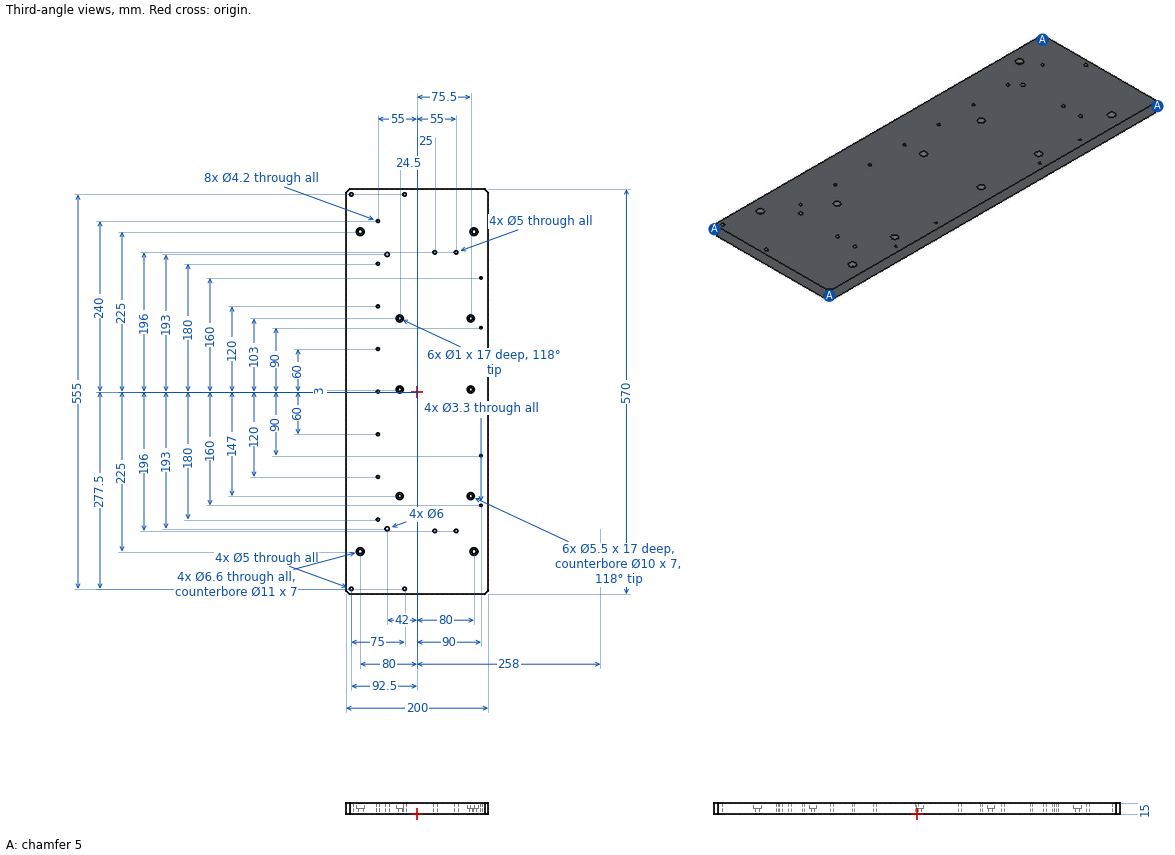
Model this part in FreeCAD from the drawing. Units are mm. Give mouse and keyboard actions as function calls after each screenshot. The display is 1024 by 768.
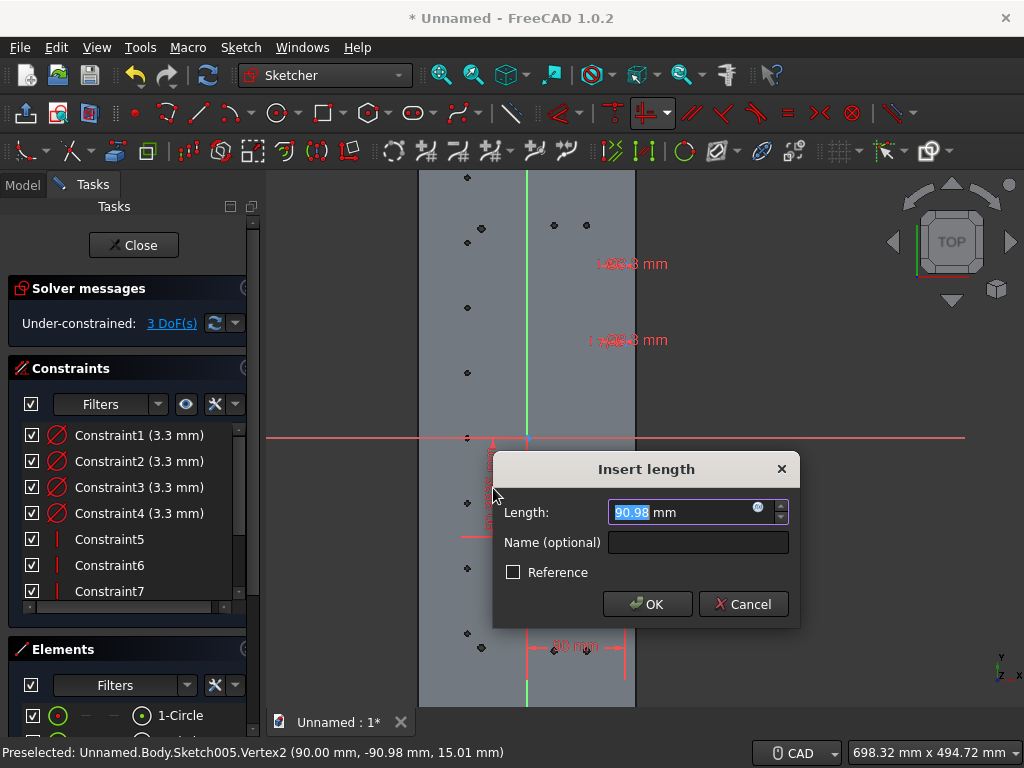
text(90)
key(Return)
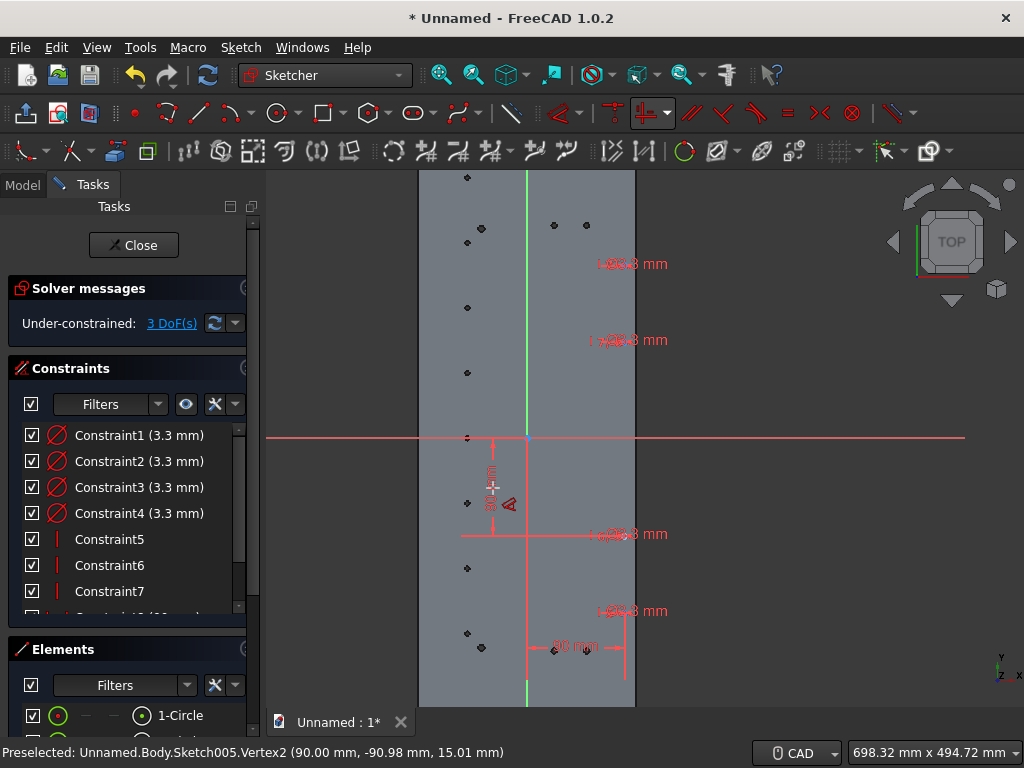
click(625, 342)
click(493, 390)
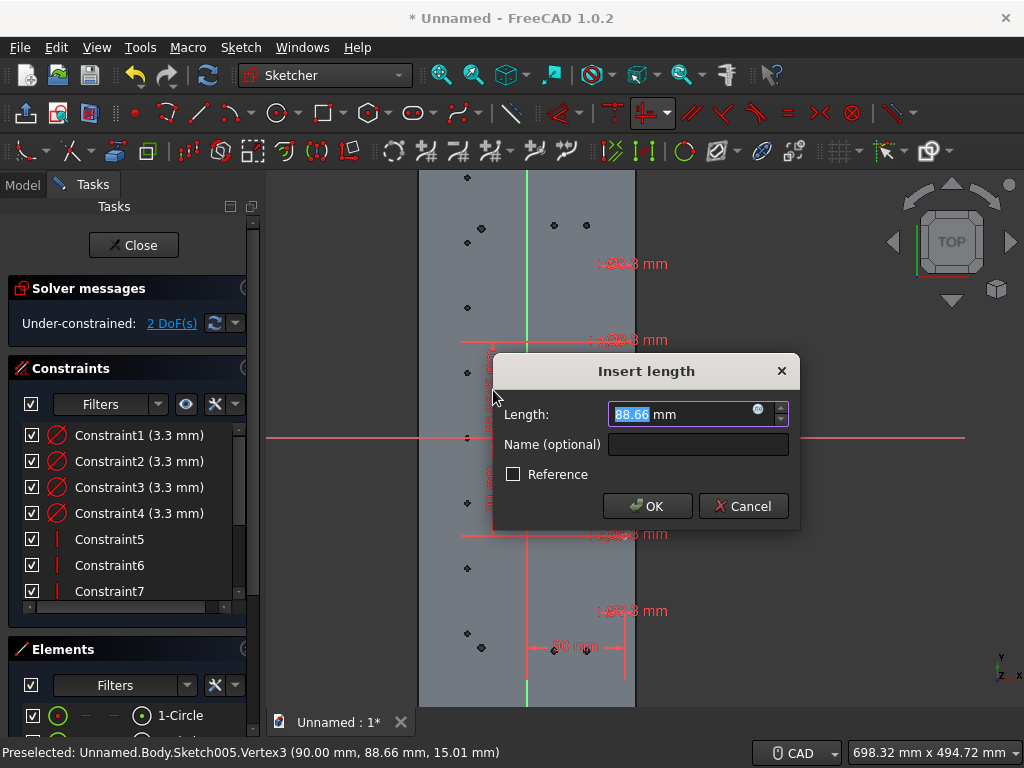
text(90)
key(Return)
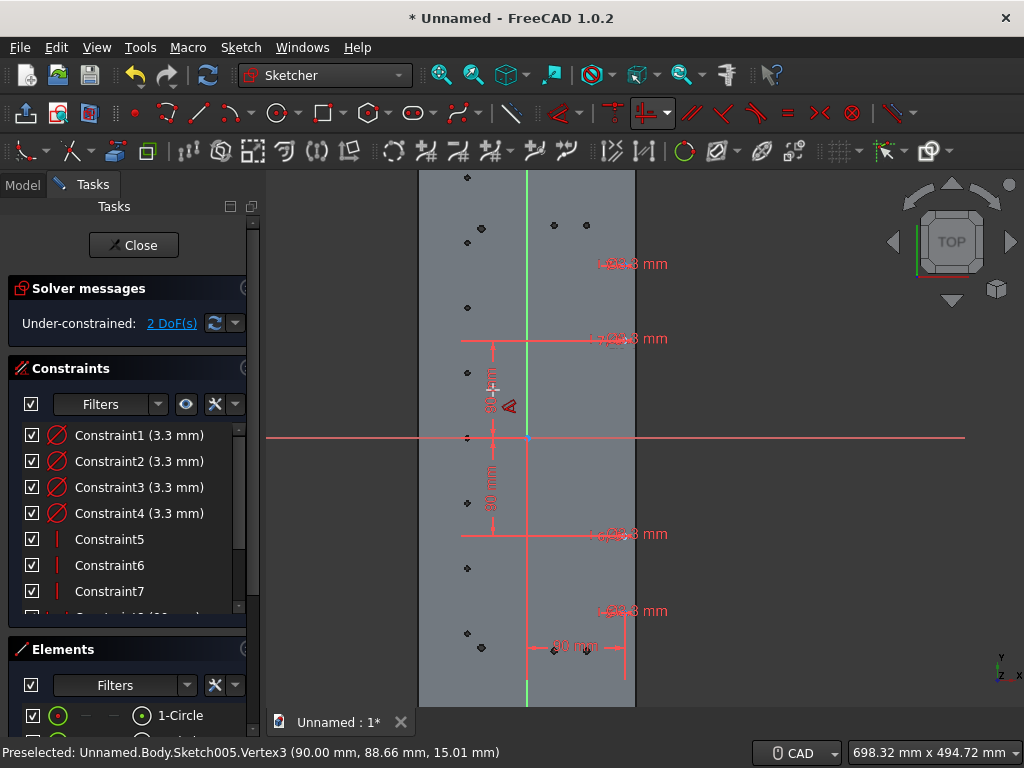
click(625, 613)
click(493, 526)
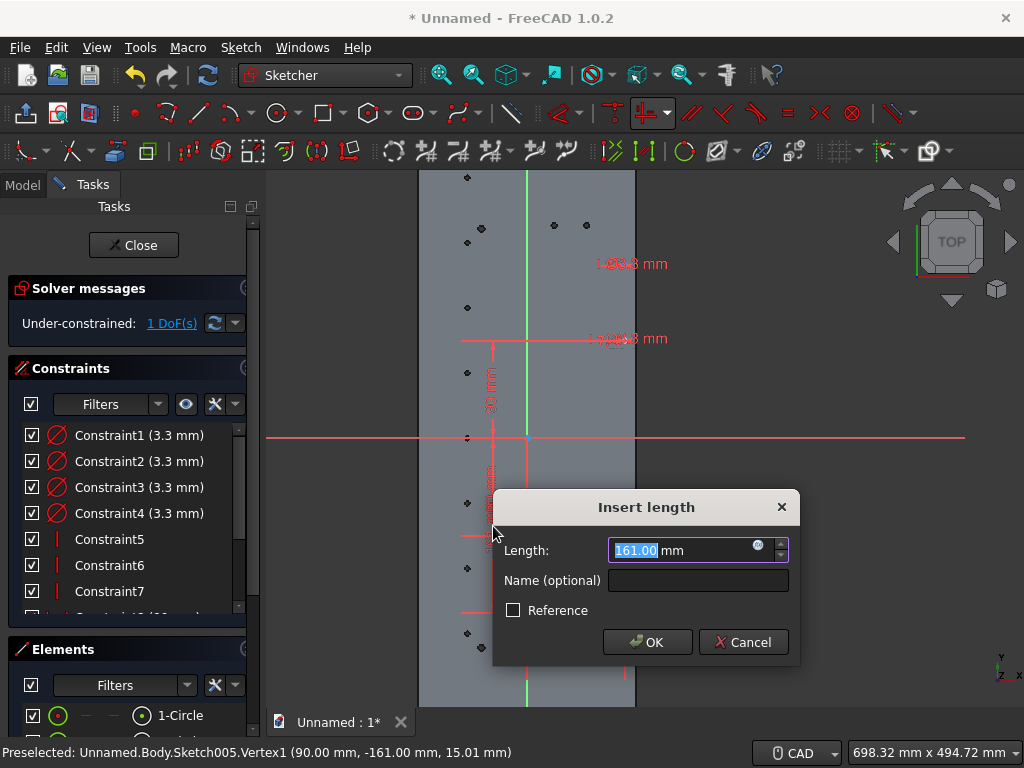
text(160)
key(Return)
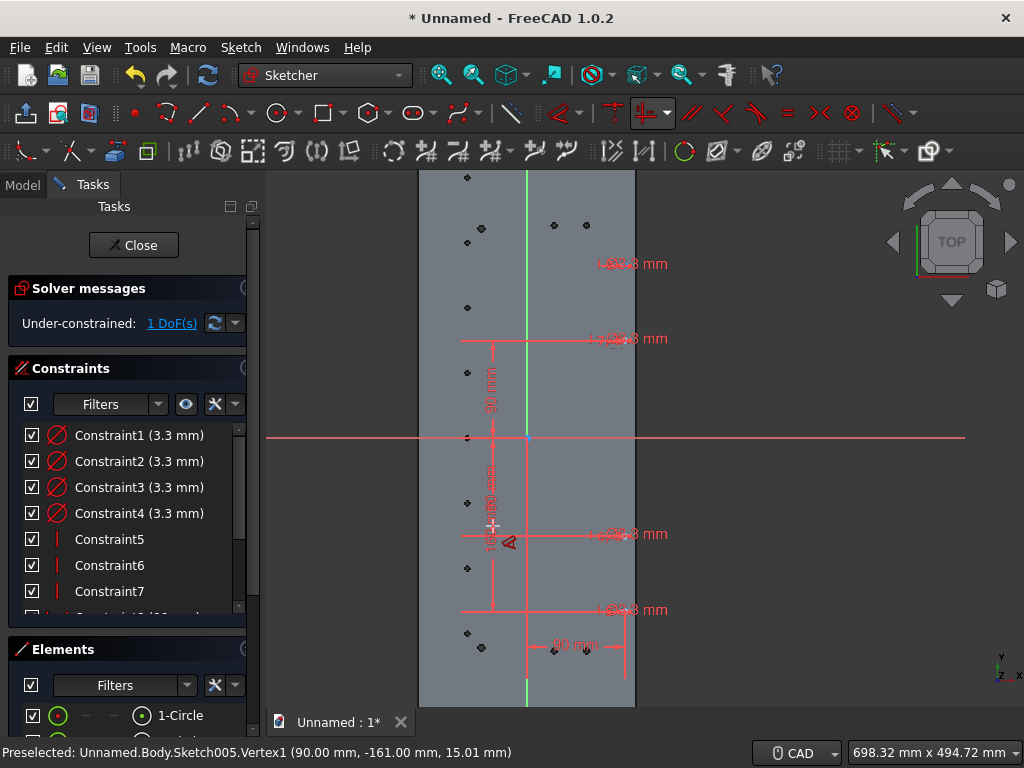
click(625, 266)
click(493, 352)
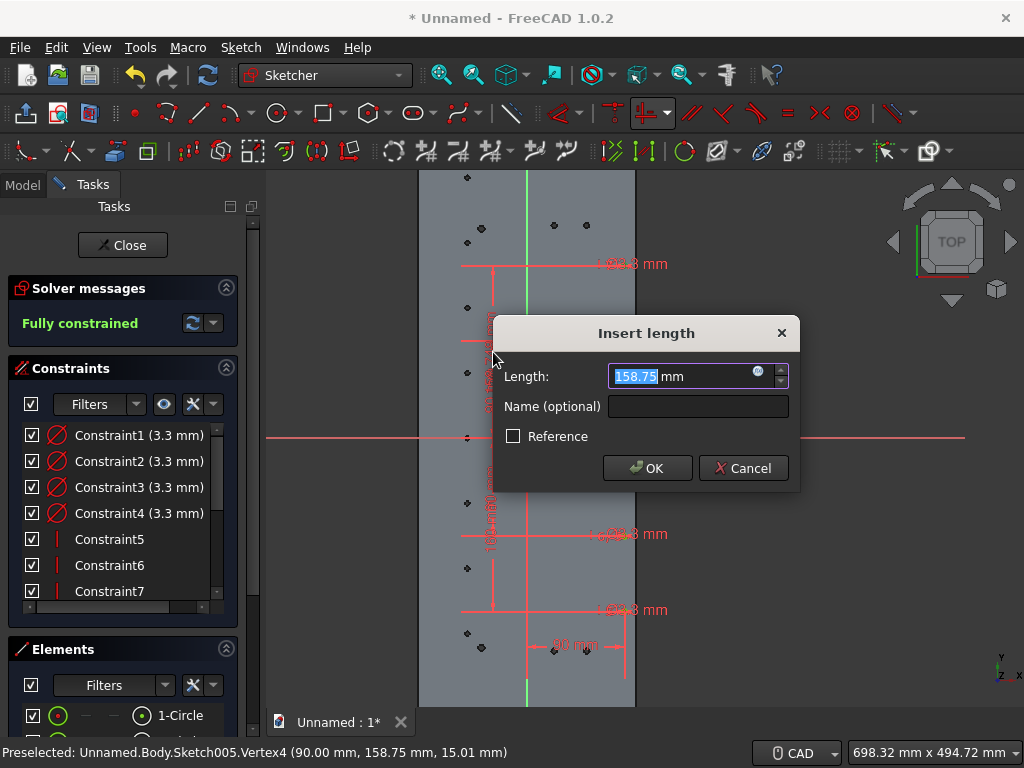
text(160)
key(Return)
key(Escape)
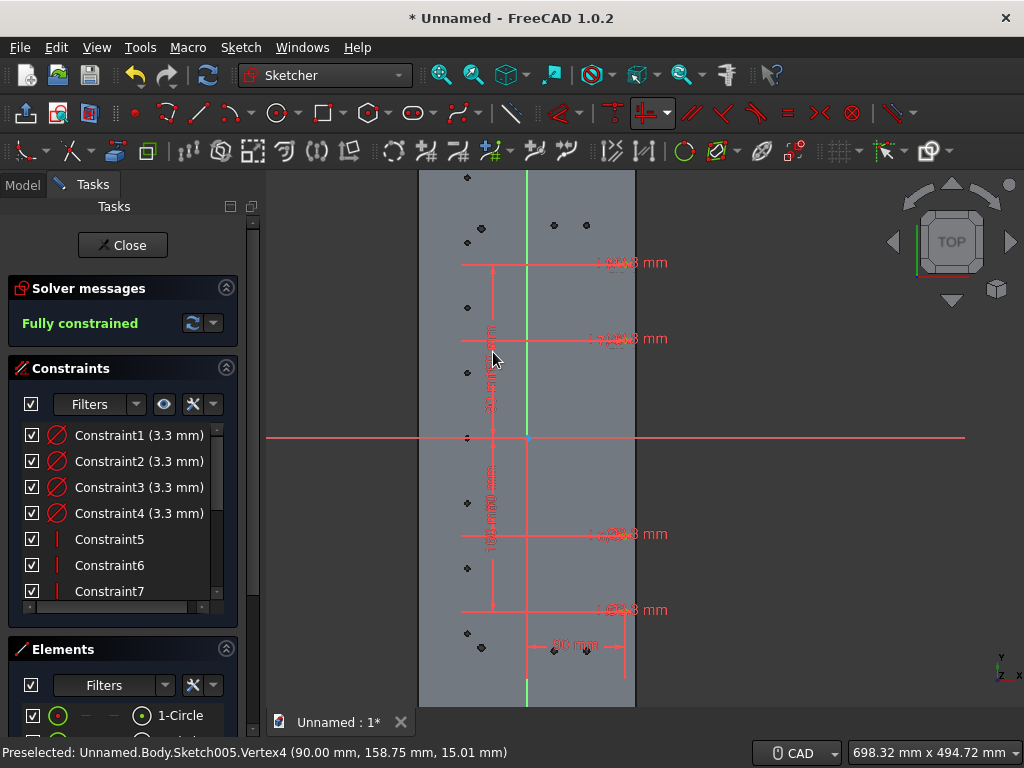
click(123, 245)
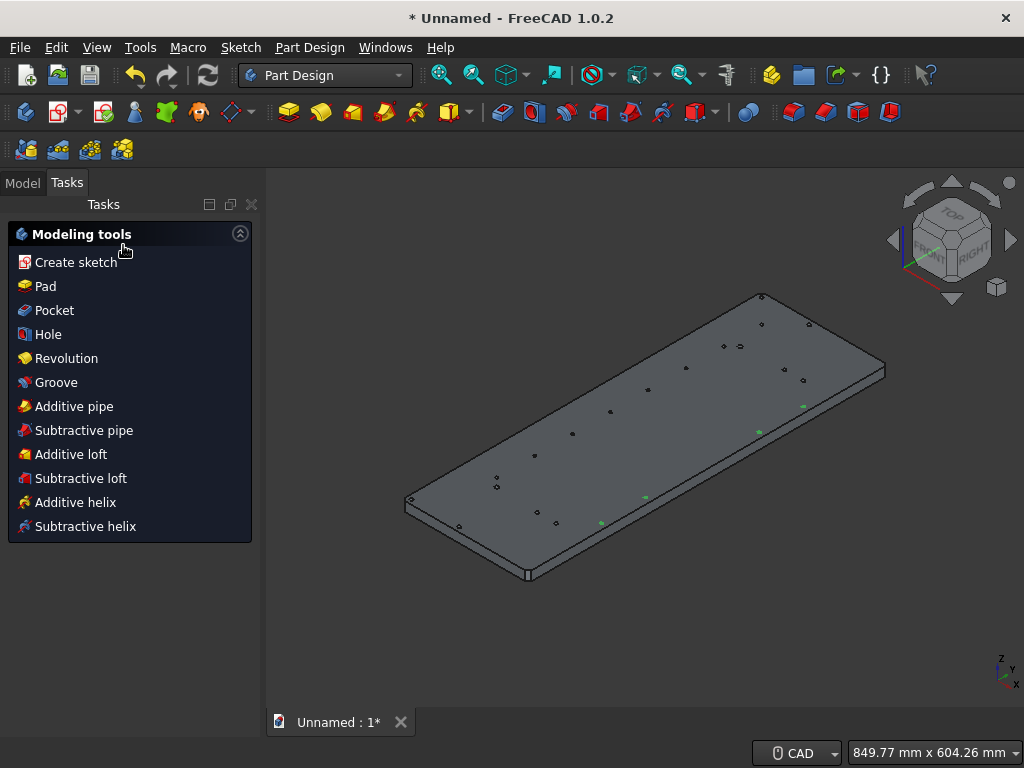
click(536, 112)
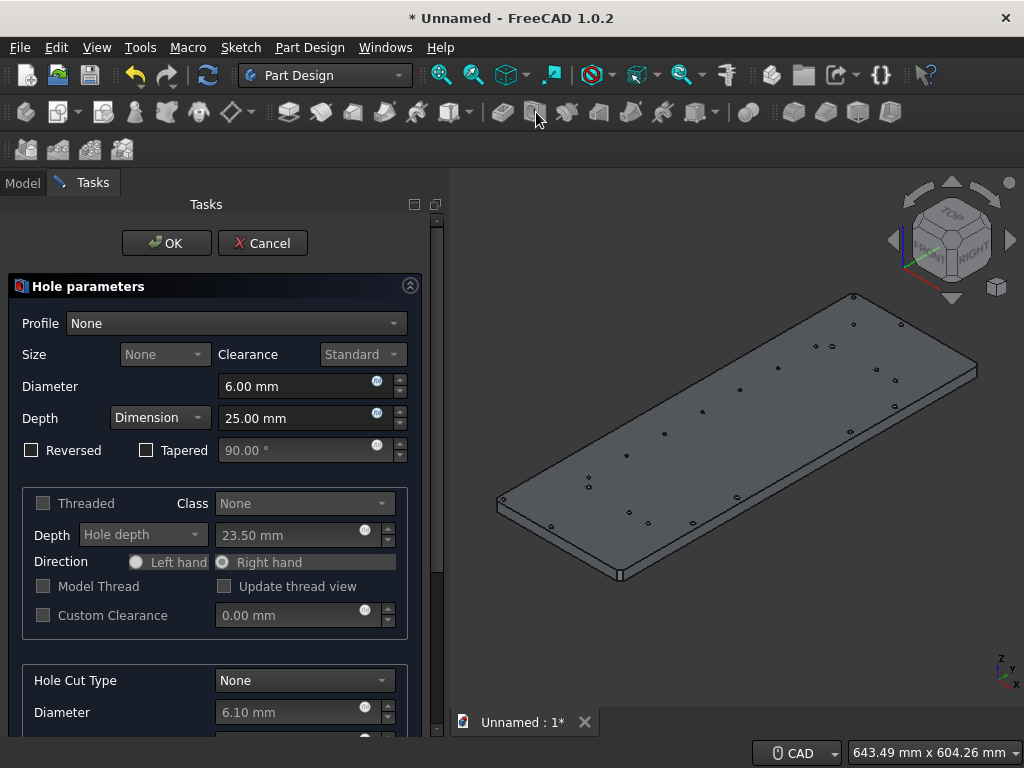
triple_click(305, 386)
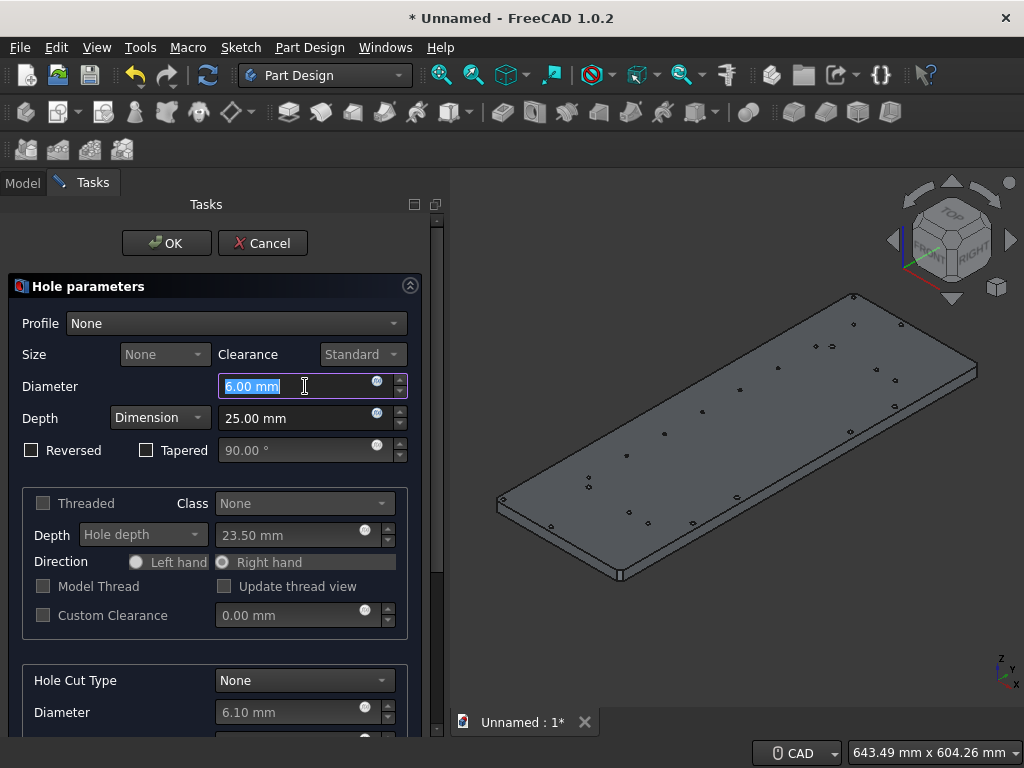
text(3.3)
key(Tab)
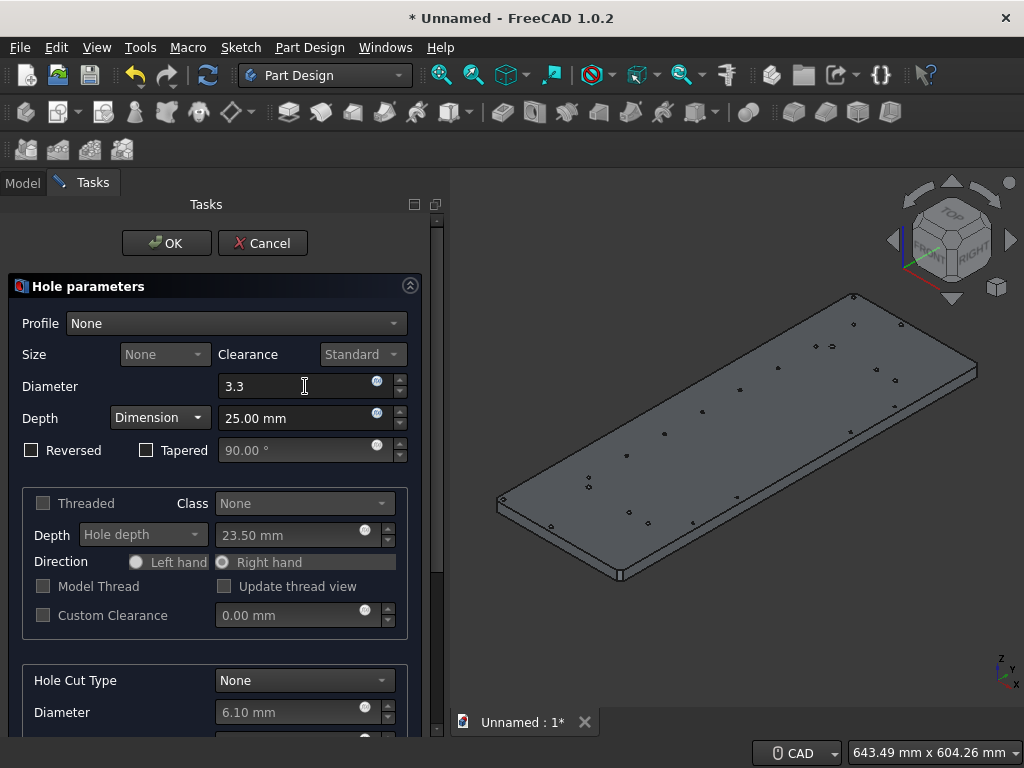
click(161, 418)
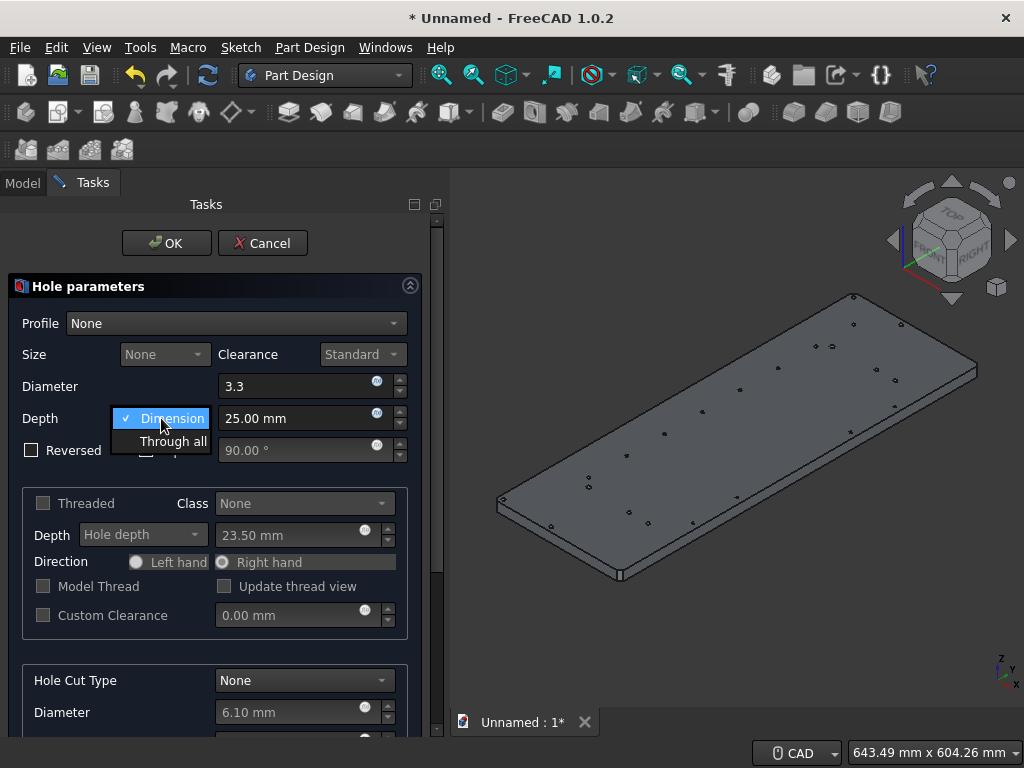
click(160, 442)